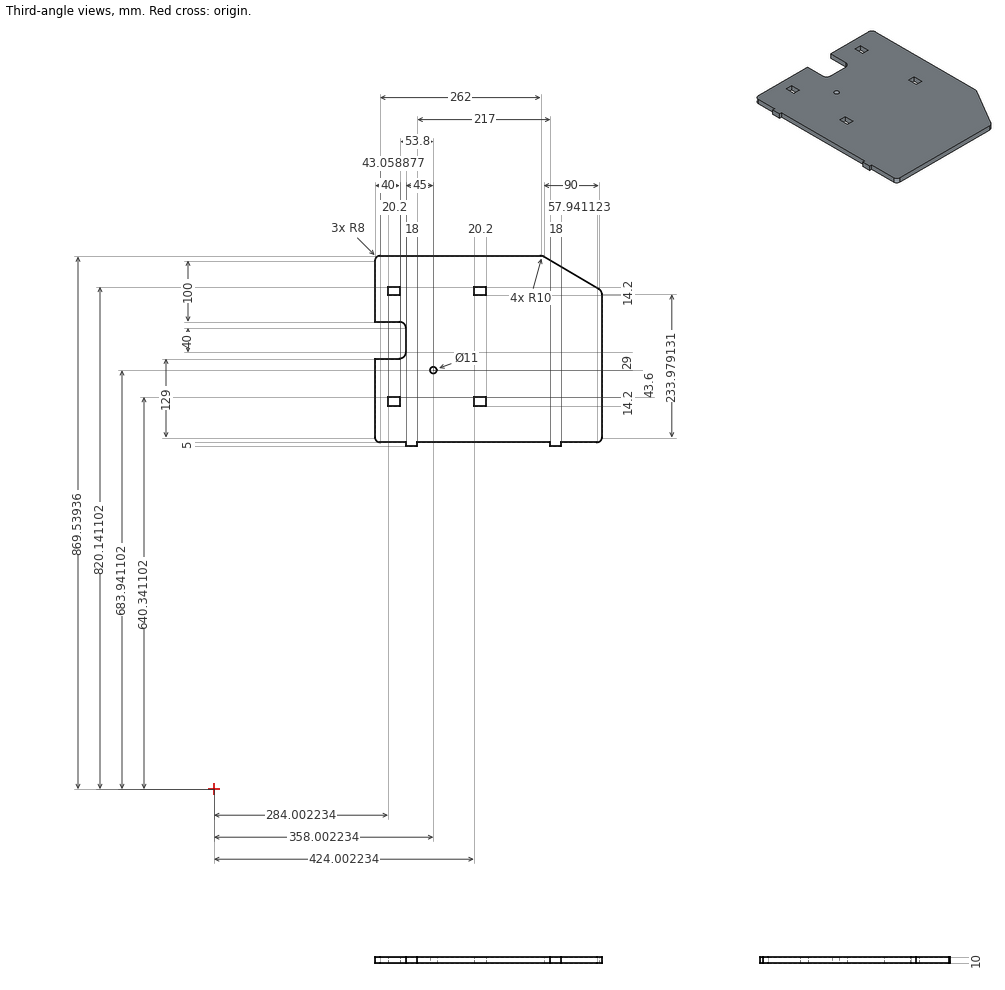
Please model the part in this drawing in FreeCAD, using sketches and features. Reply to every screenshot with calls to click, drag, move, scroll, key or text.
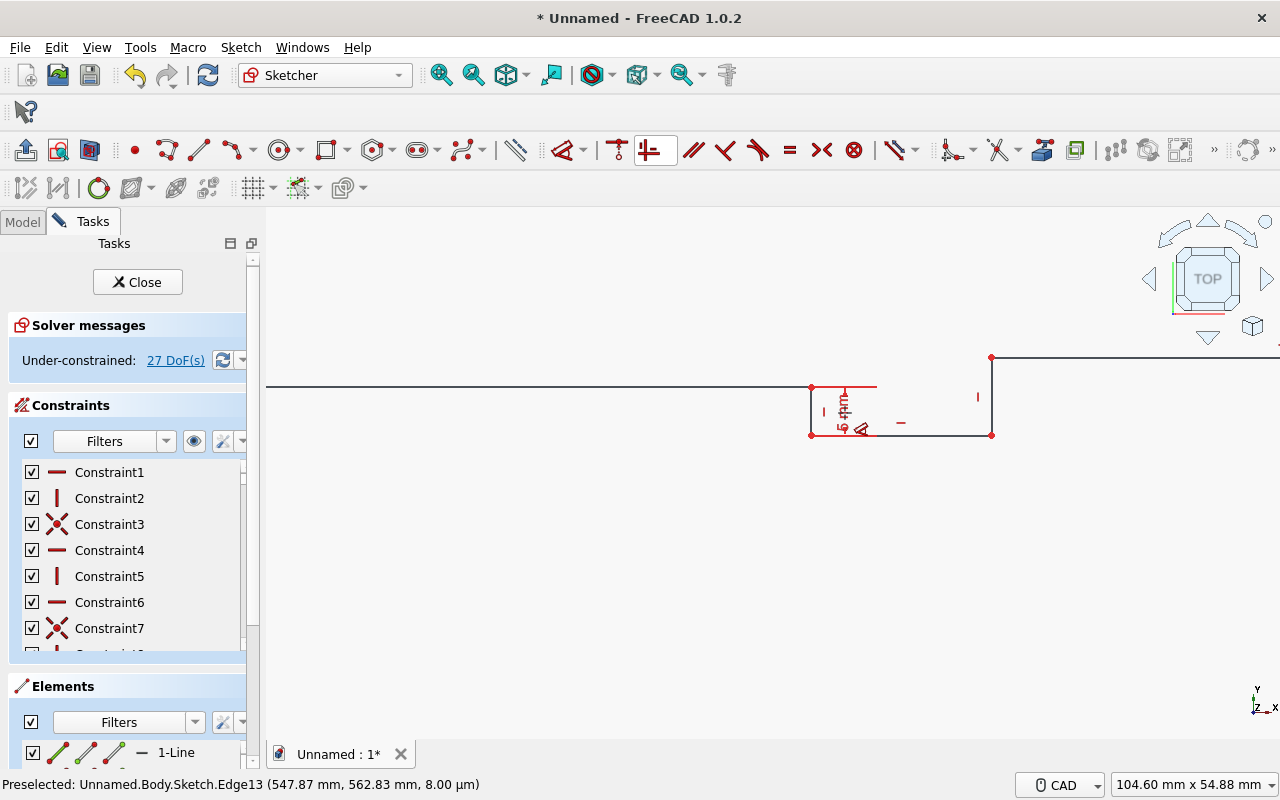
click(992, 412)
click(1026, 397)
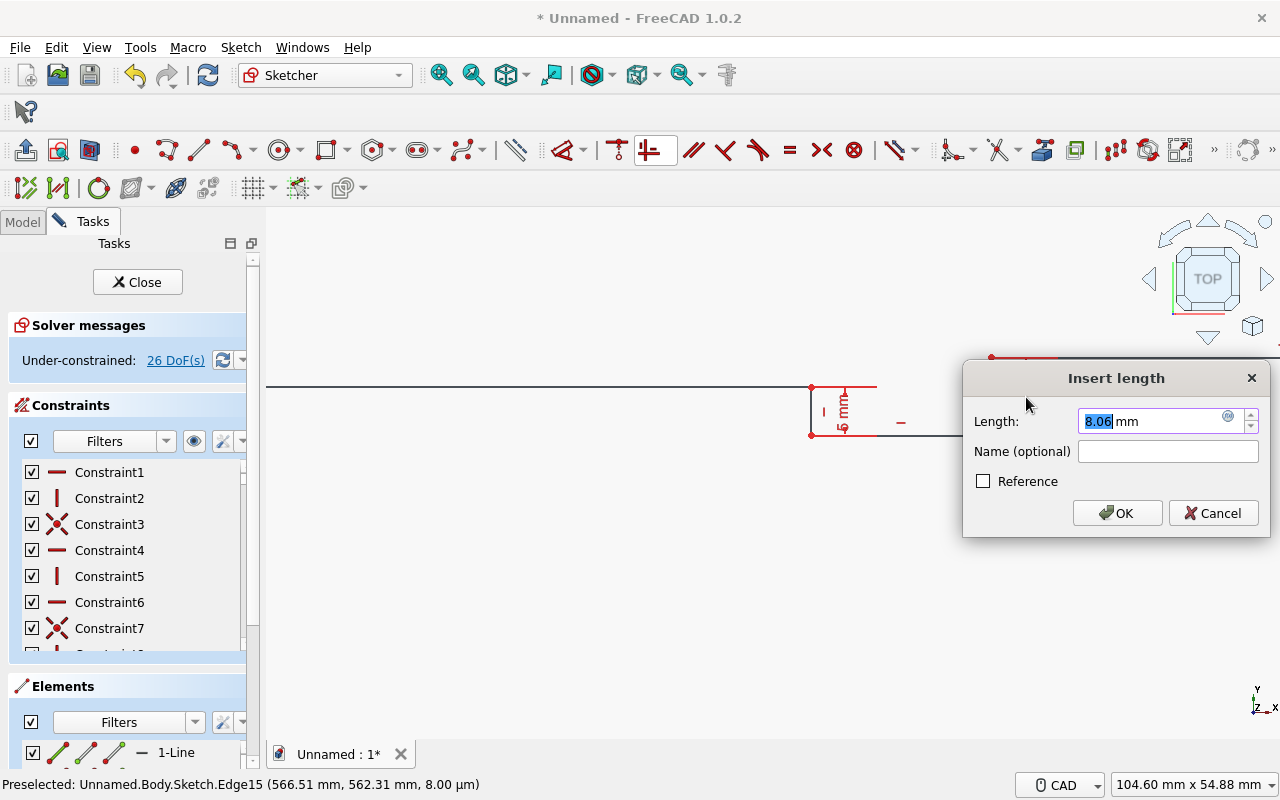
text(5)
key(Return)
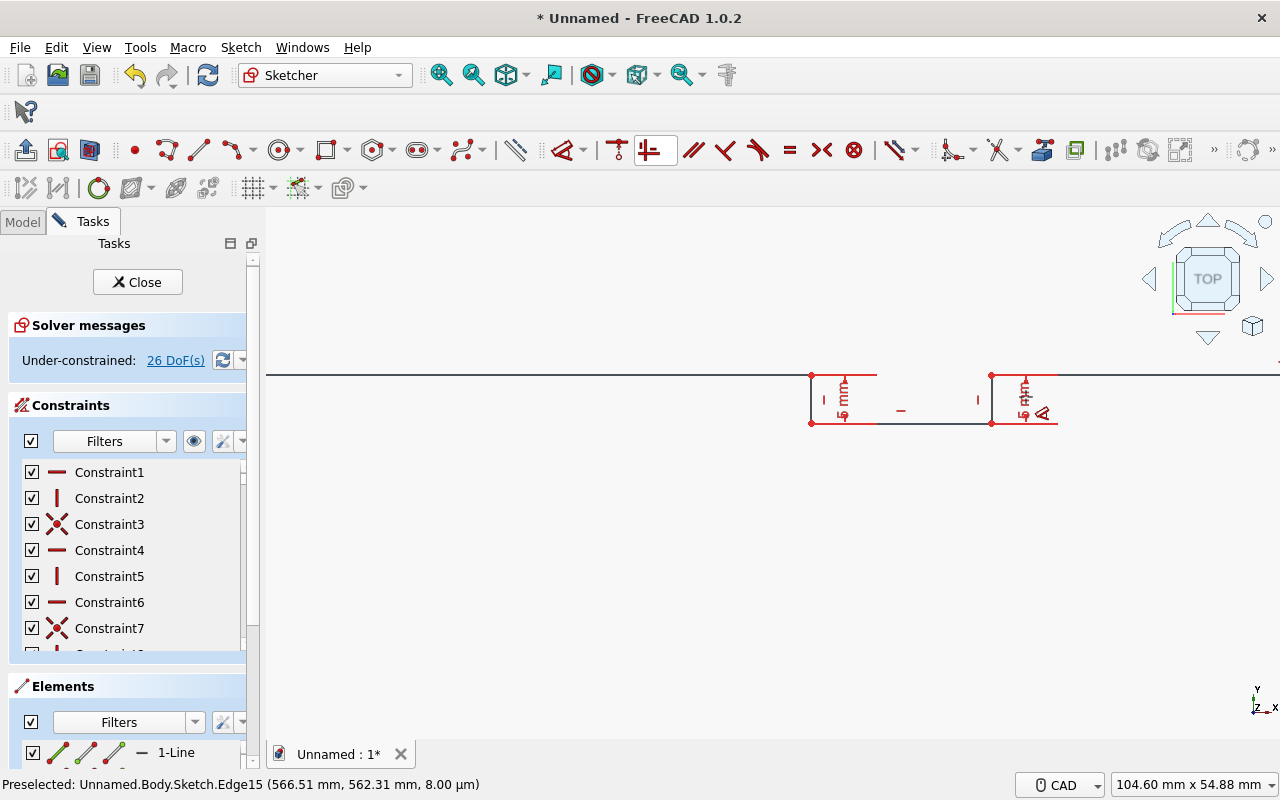
scroll(816, 412, down, 15)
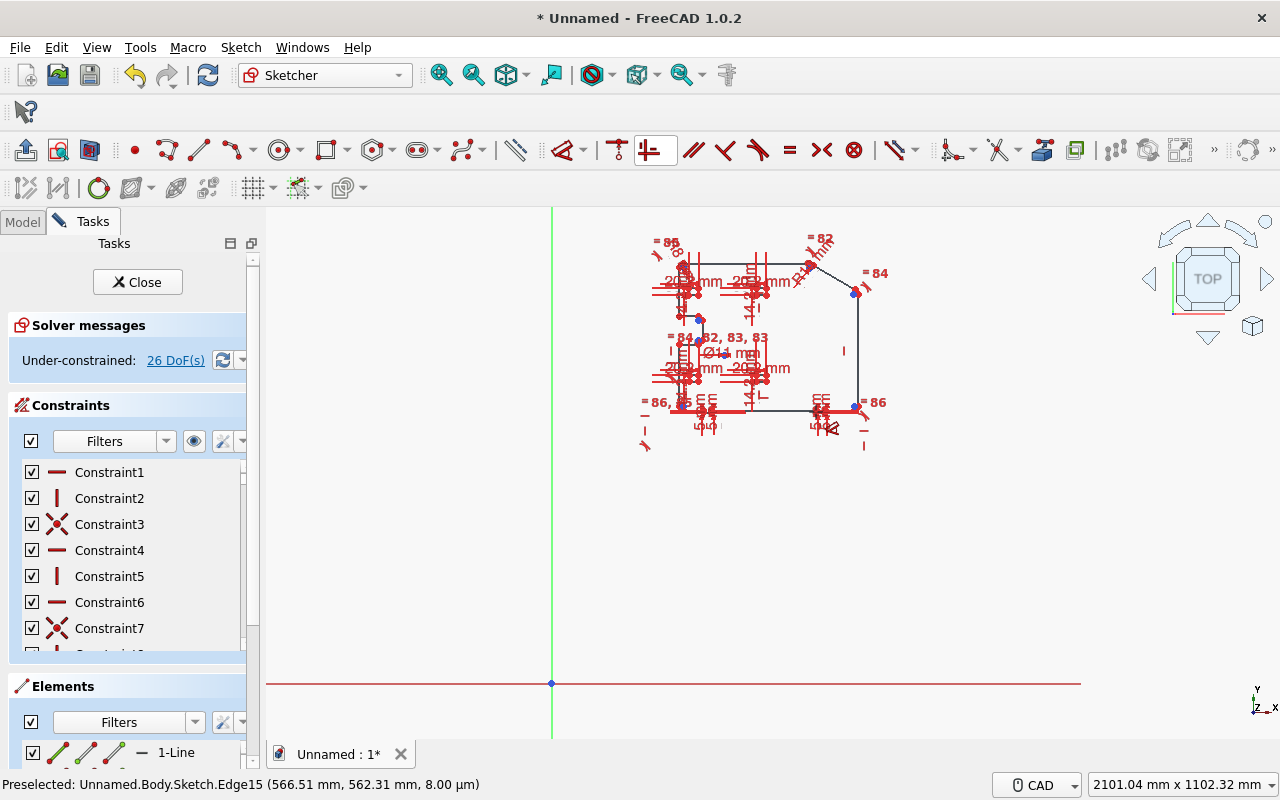
scroll(685, 316, up, 5)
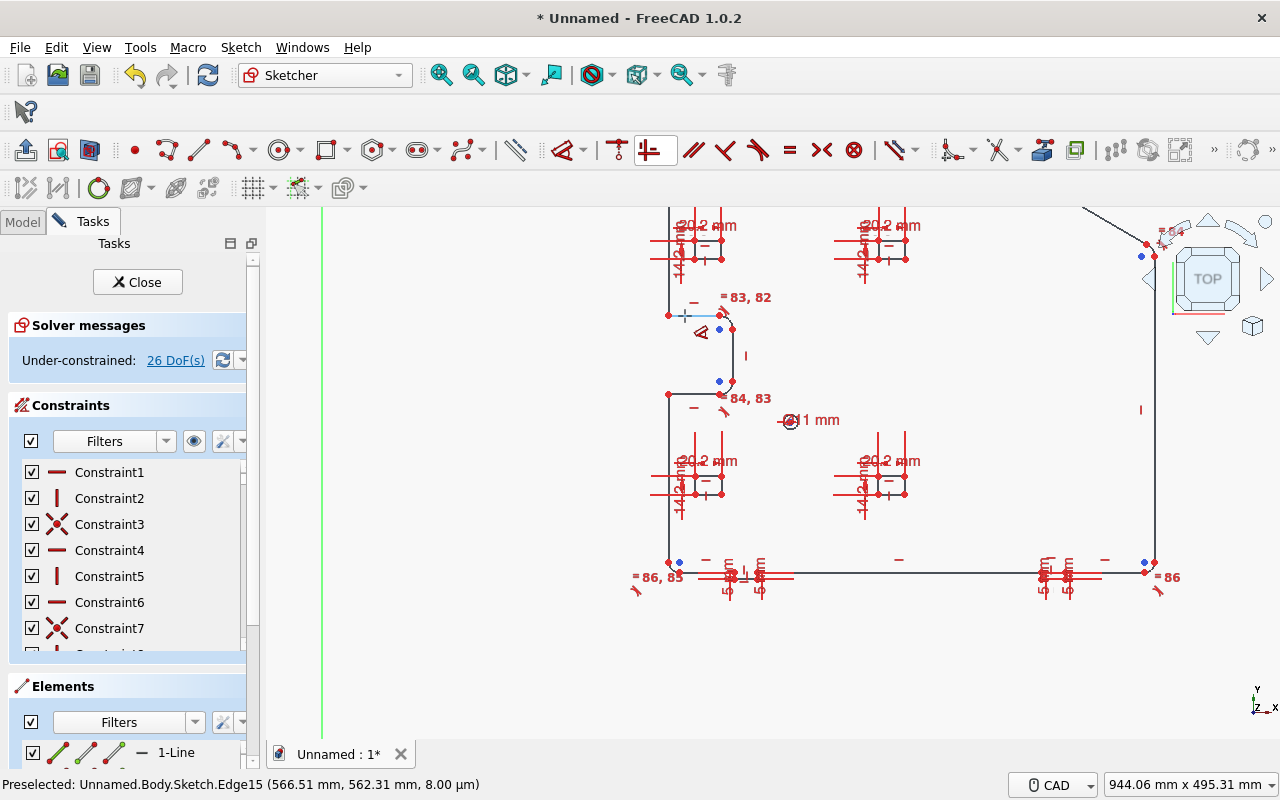
click(684, 316)
click(694, 282)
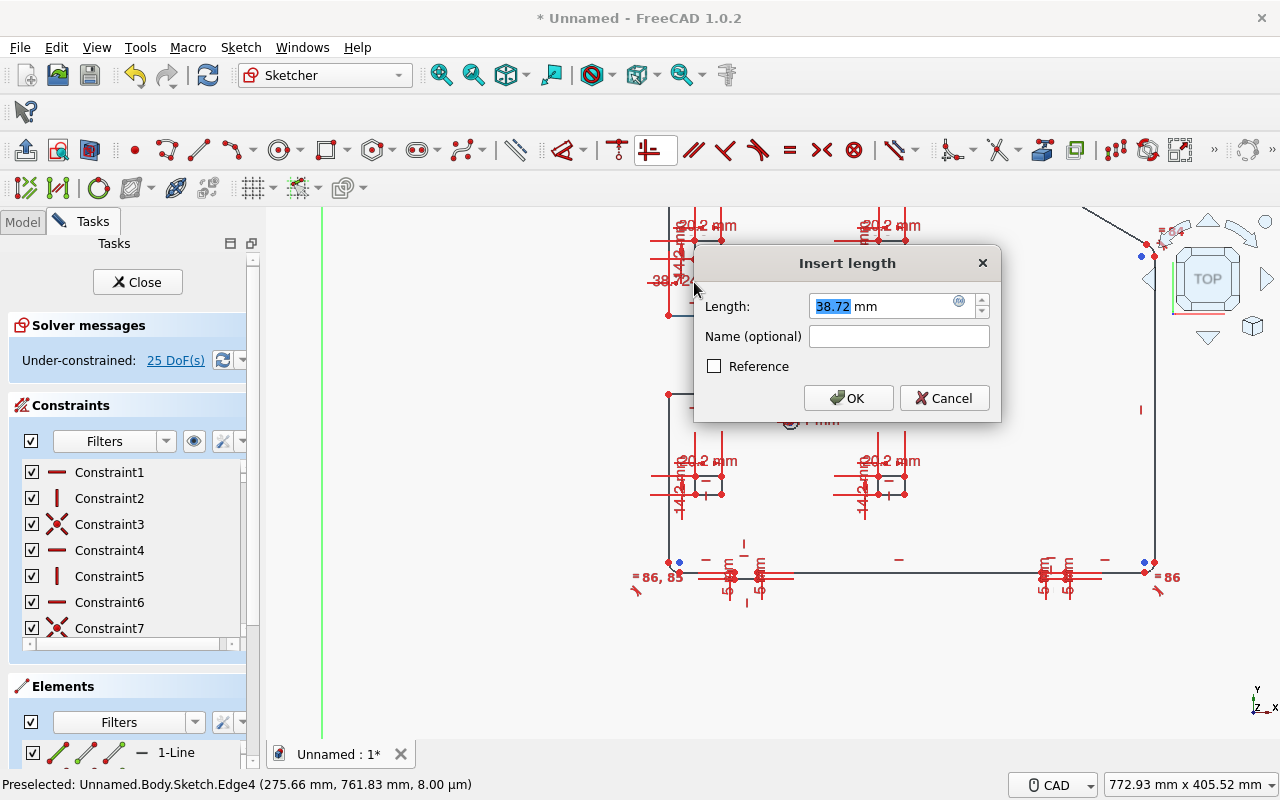
text(40)
key(Return)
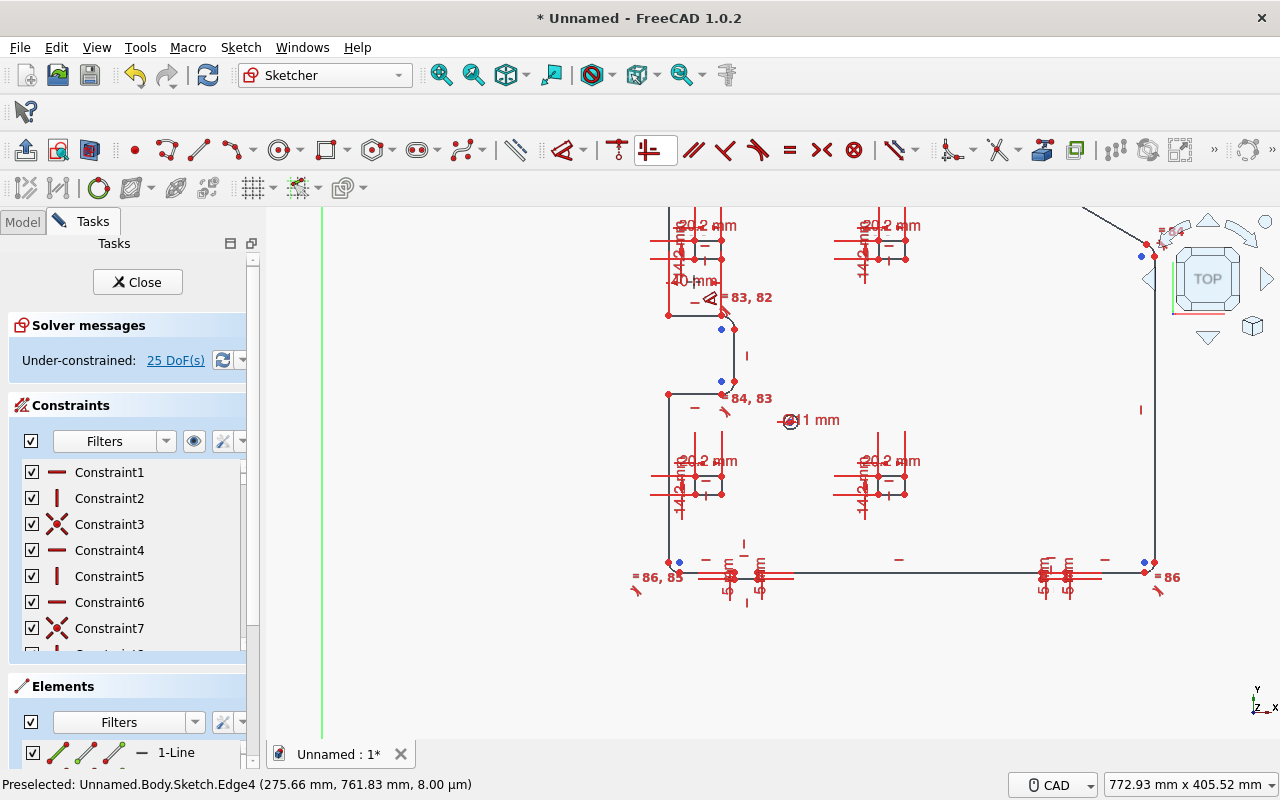
click(734, 345)
click(700, 355)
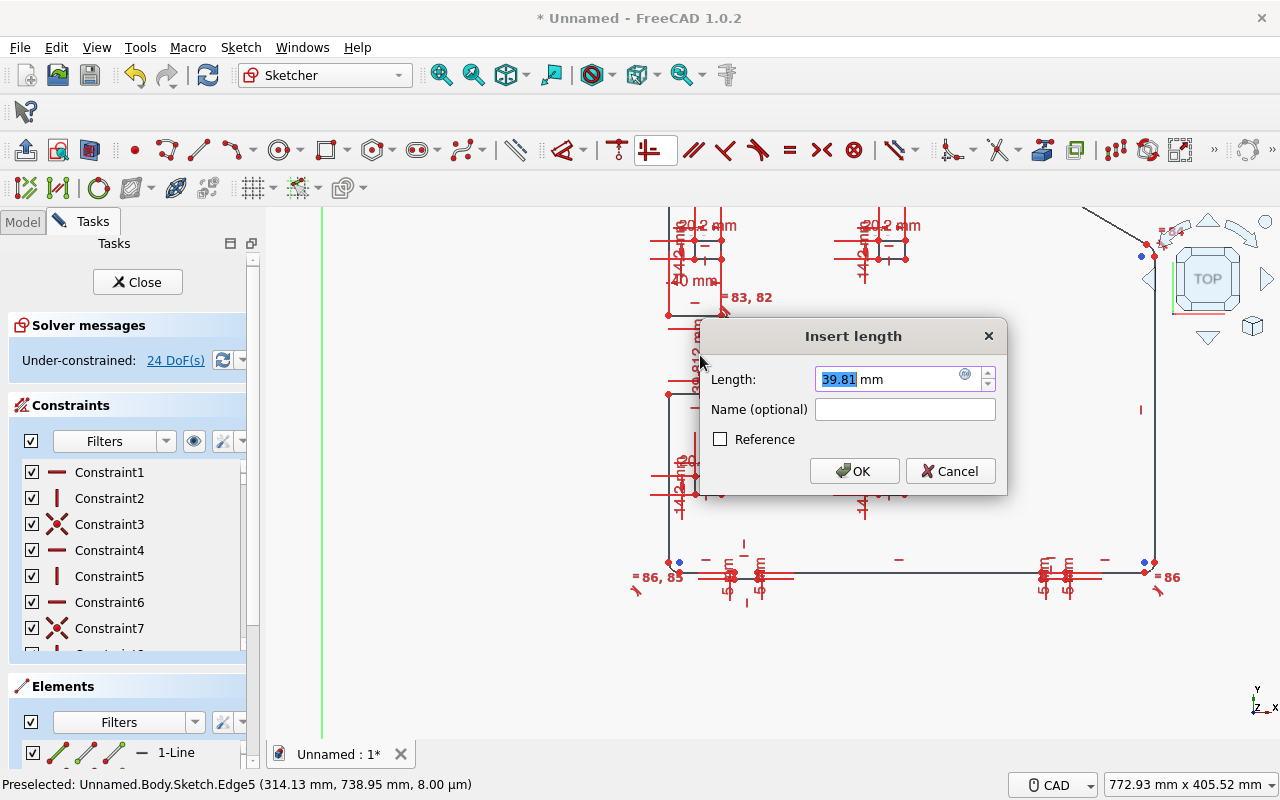
text(40)
key(Return)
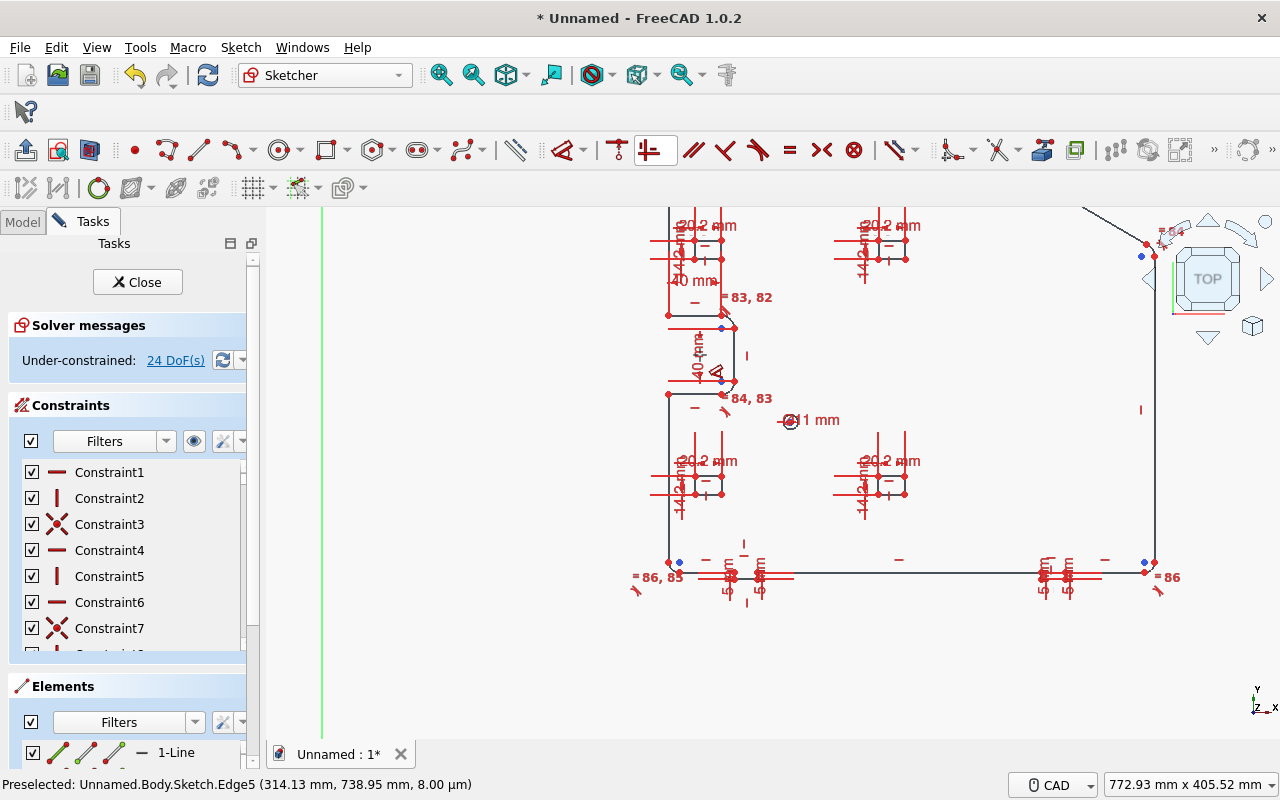
click(706, 394)
click(695, 428)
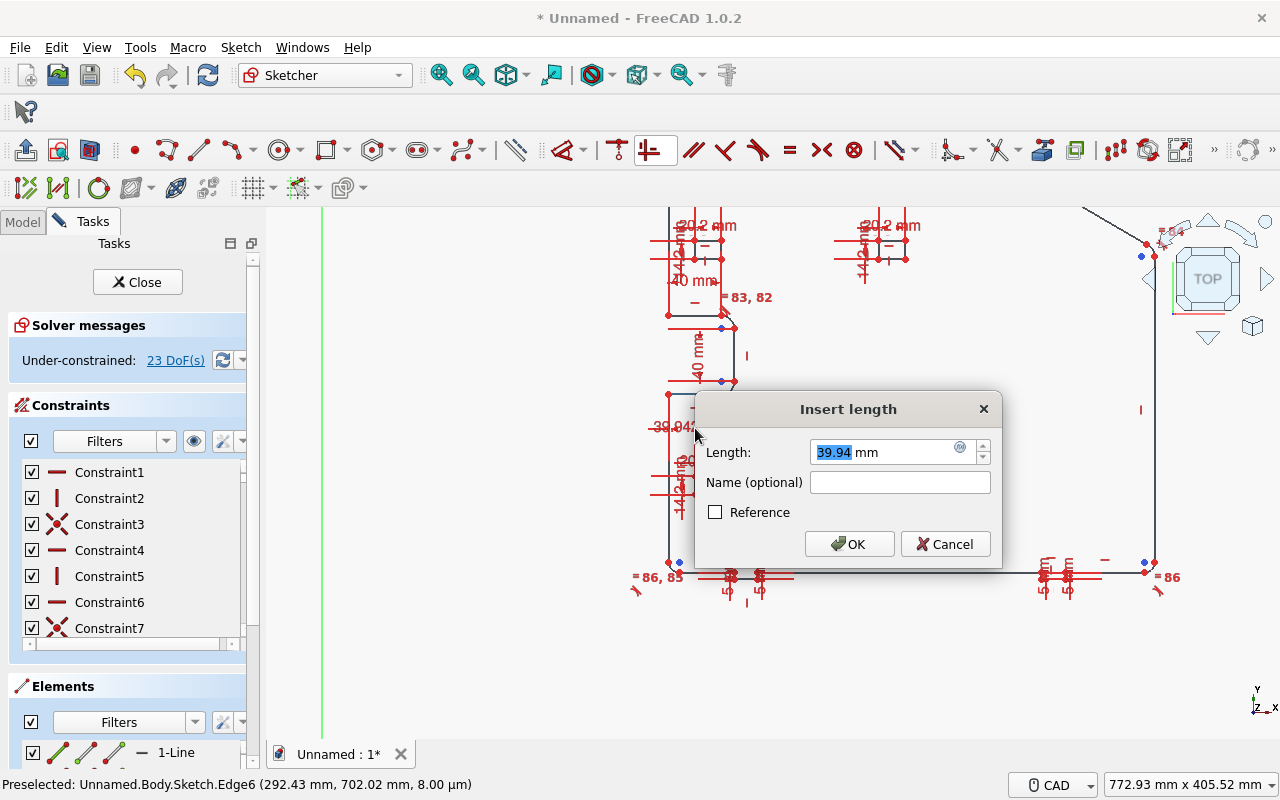
text(40)
key(Return)